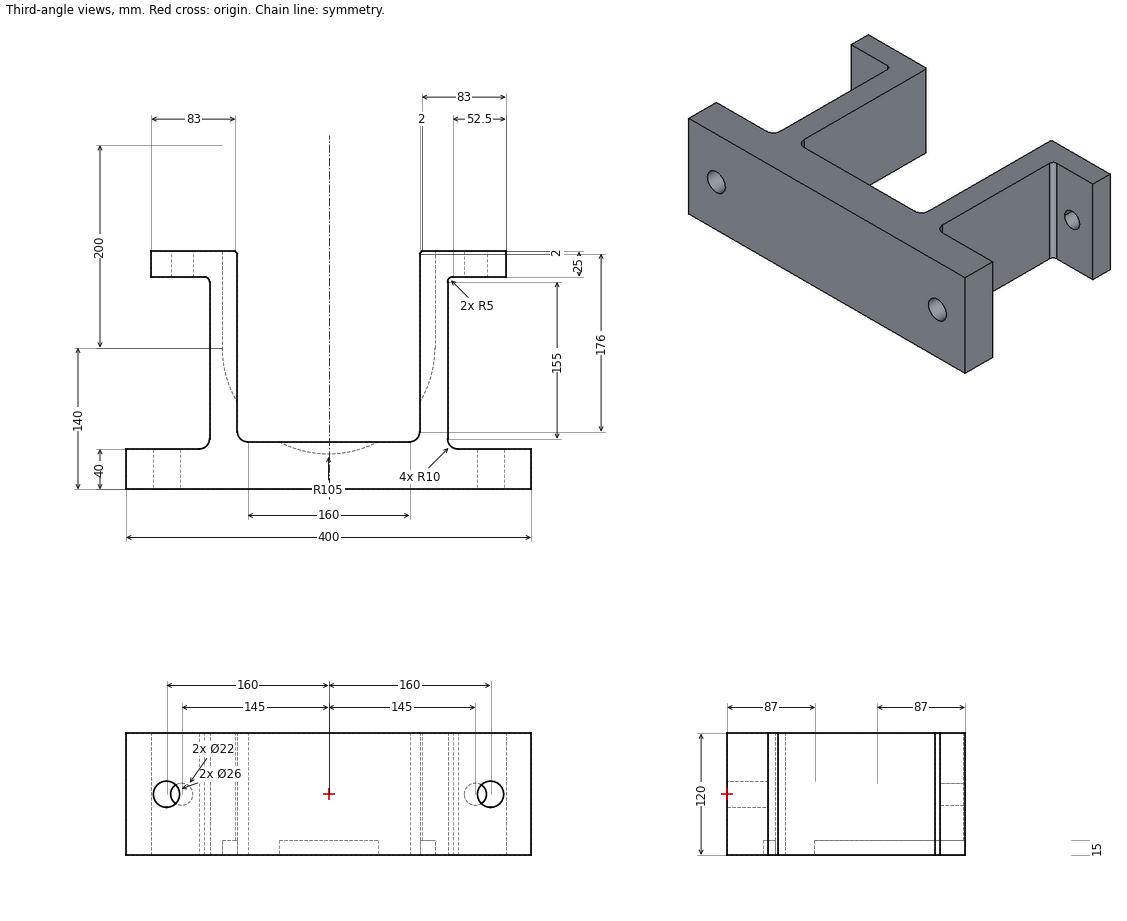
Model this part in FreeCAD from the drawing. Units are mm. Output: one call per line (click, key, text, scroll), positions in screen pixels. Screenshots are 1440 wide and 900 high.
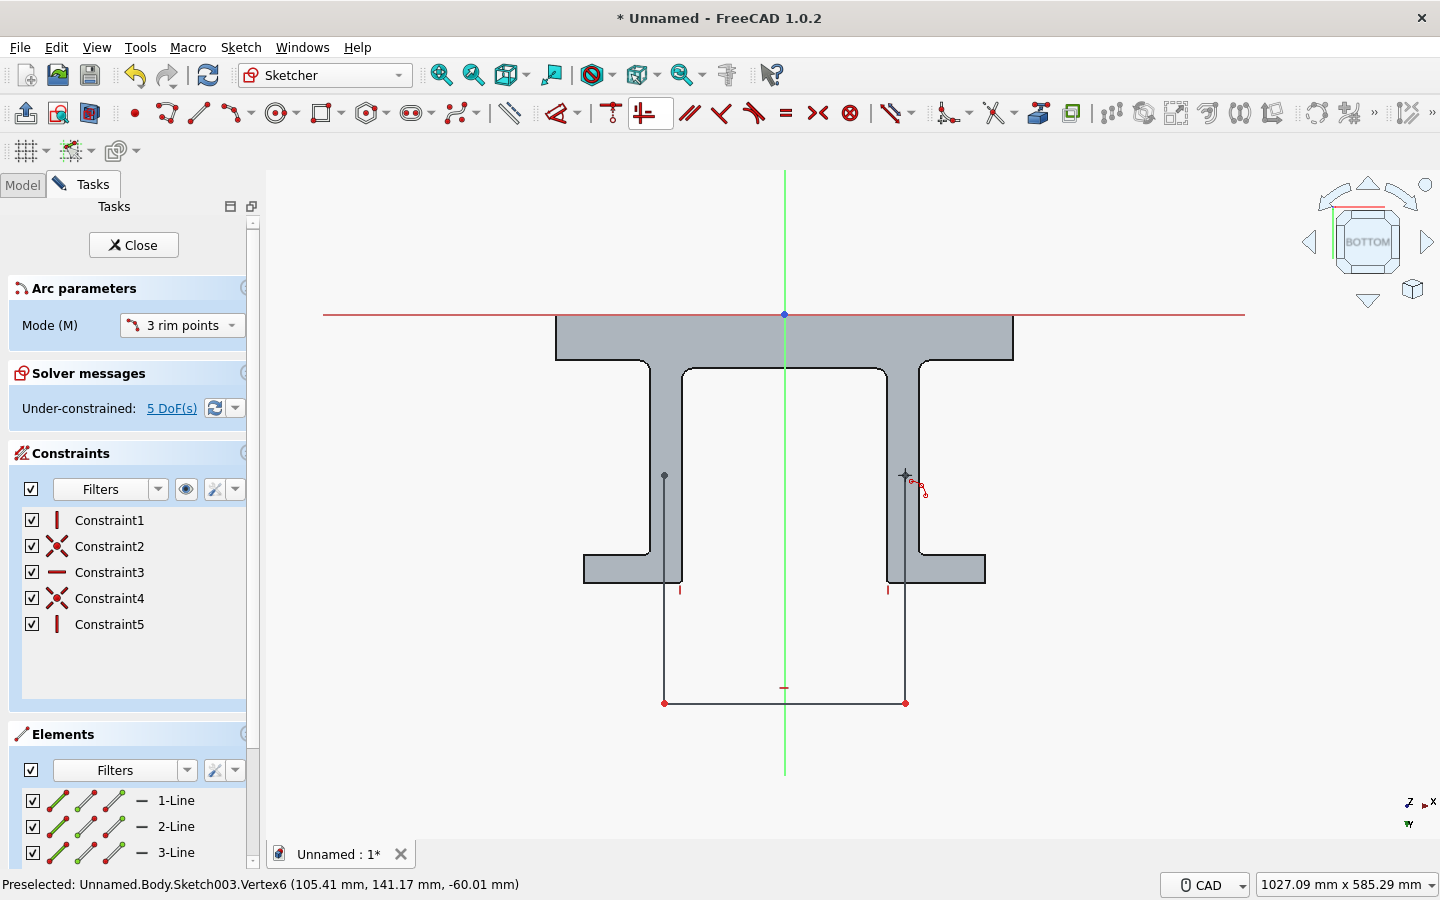
click(905, 476)
click(664, 476)
click(822, 361)
key(Escape)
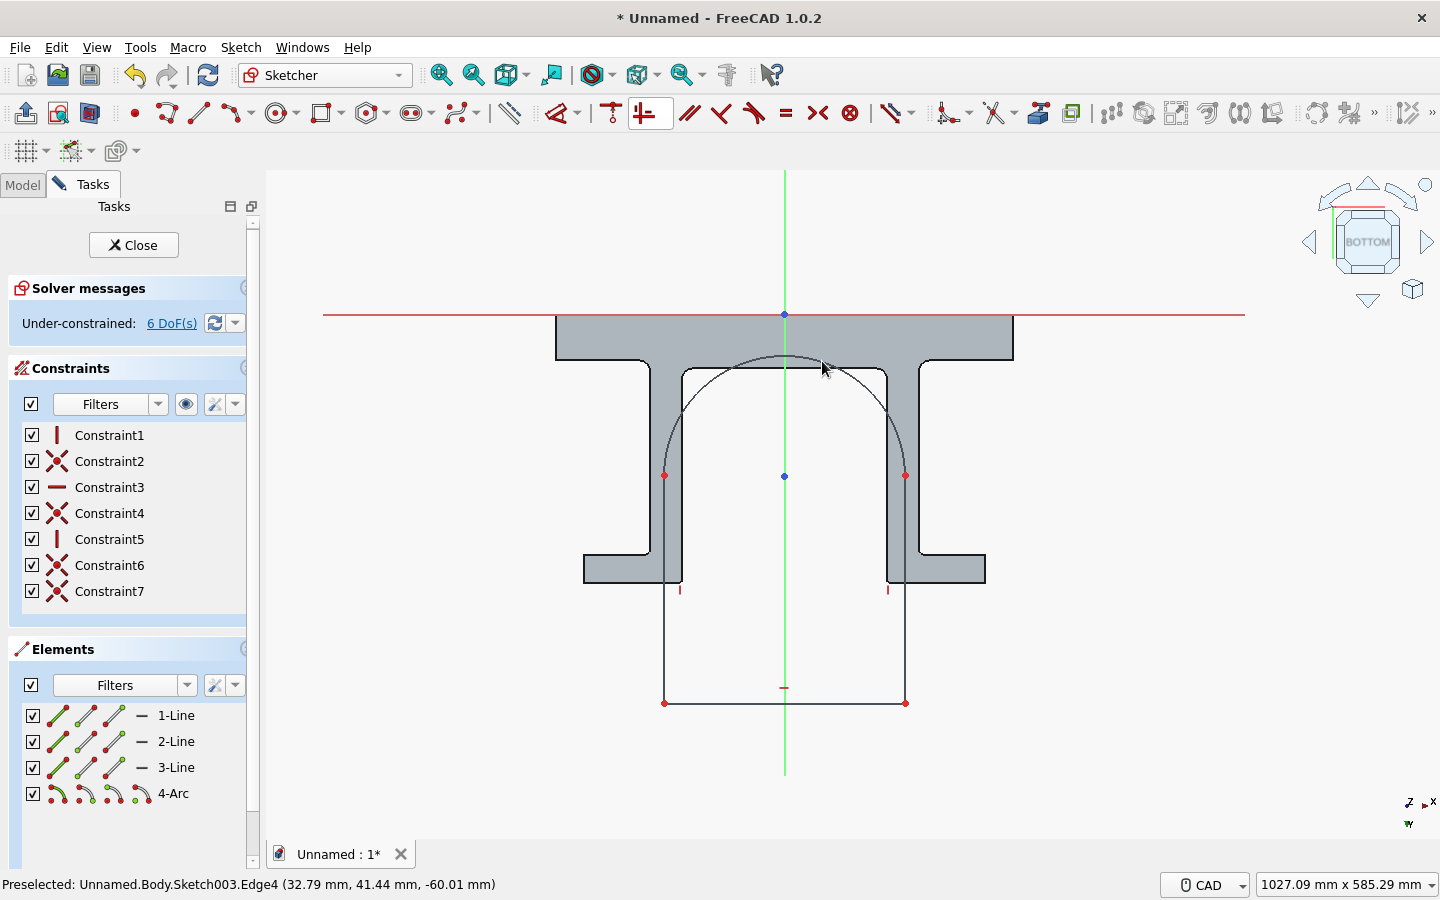
click(784, 477)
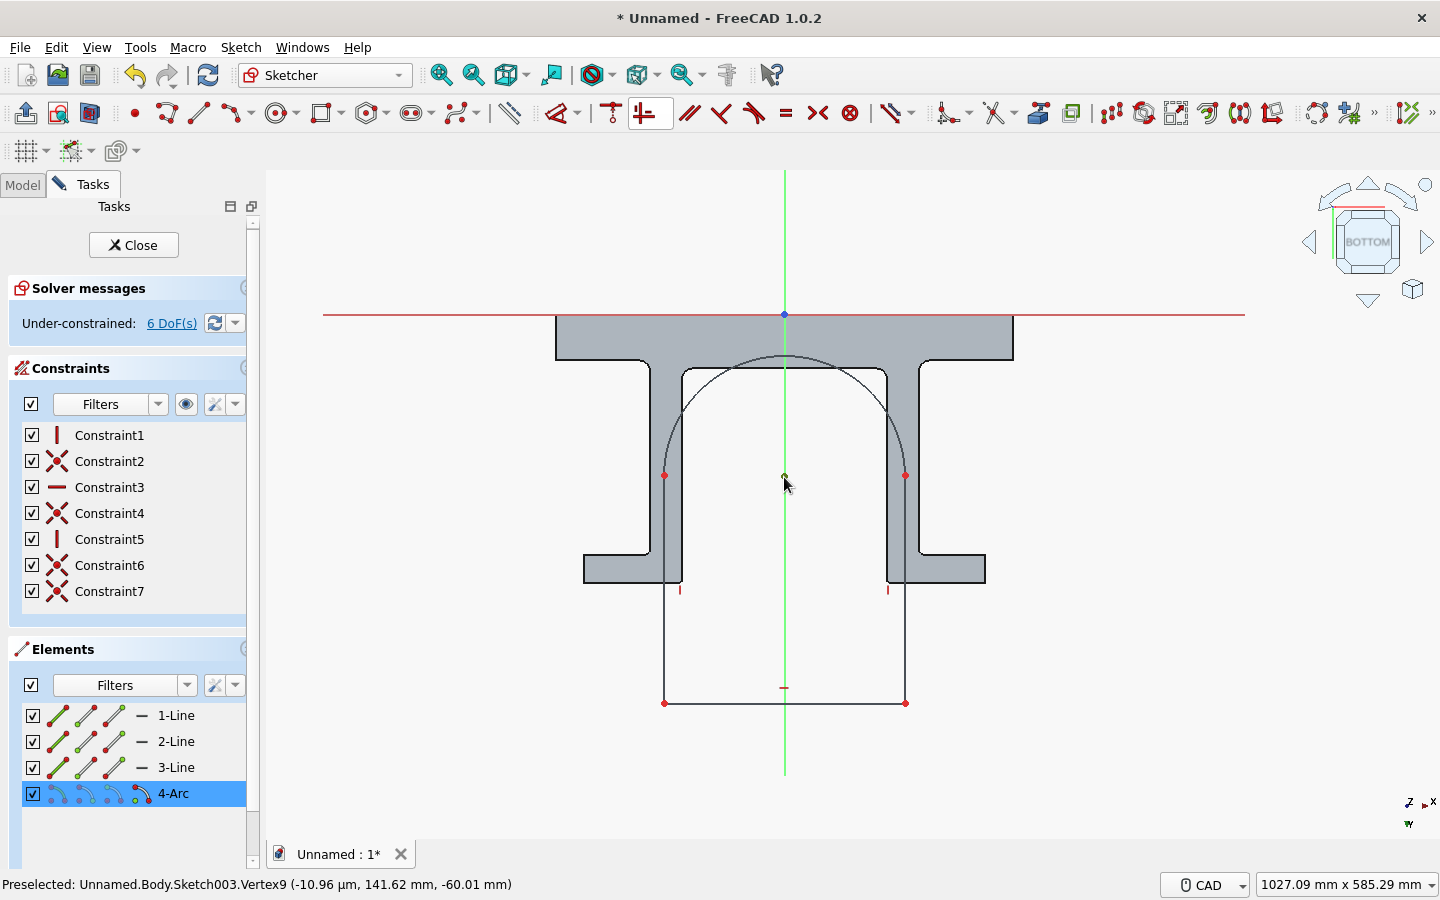
click(785, 767)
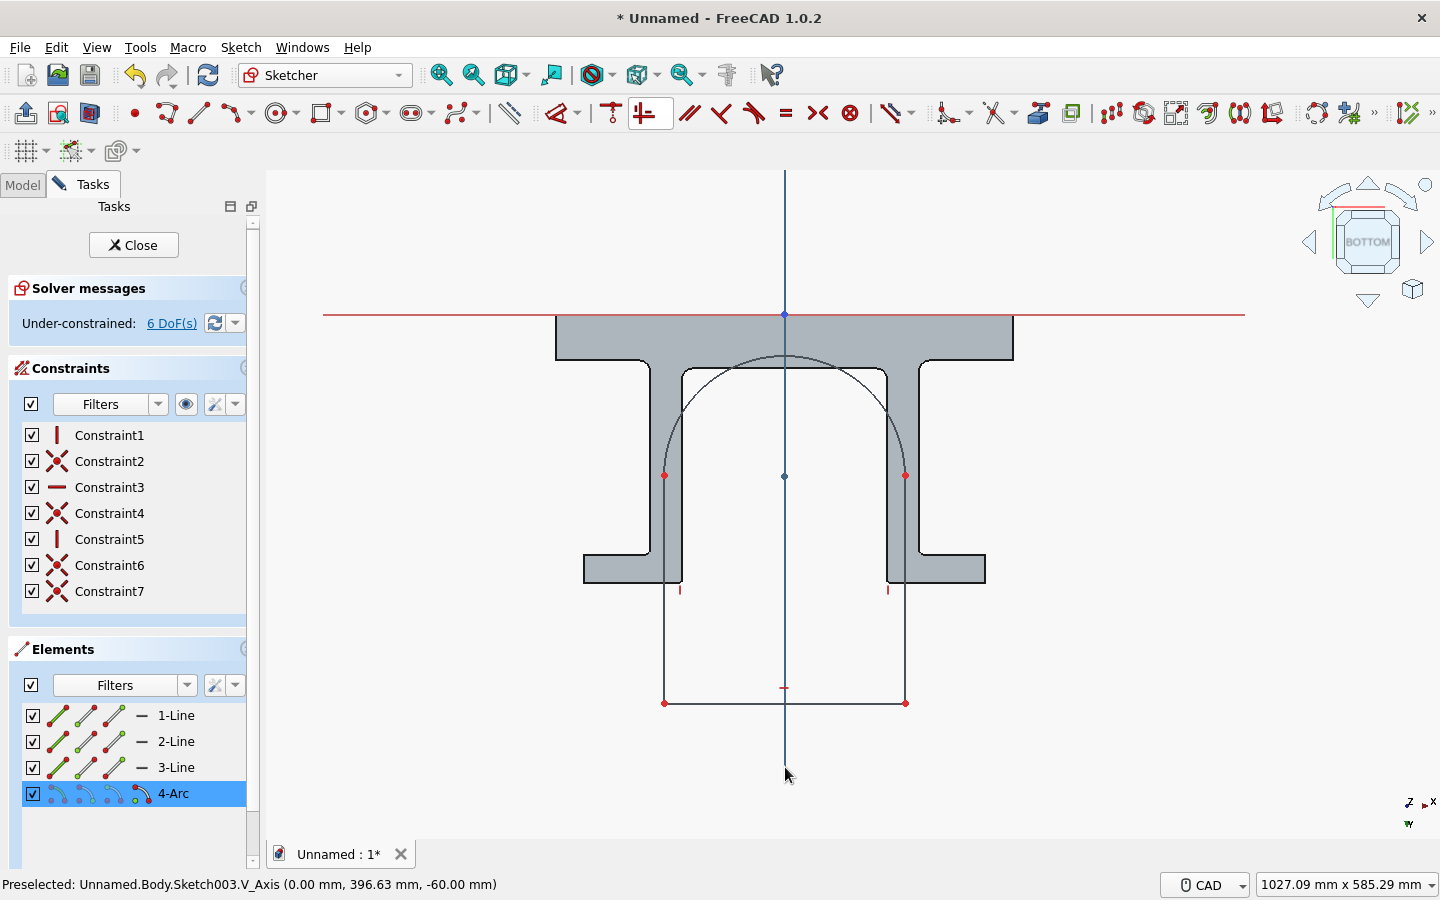
click(612, 114)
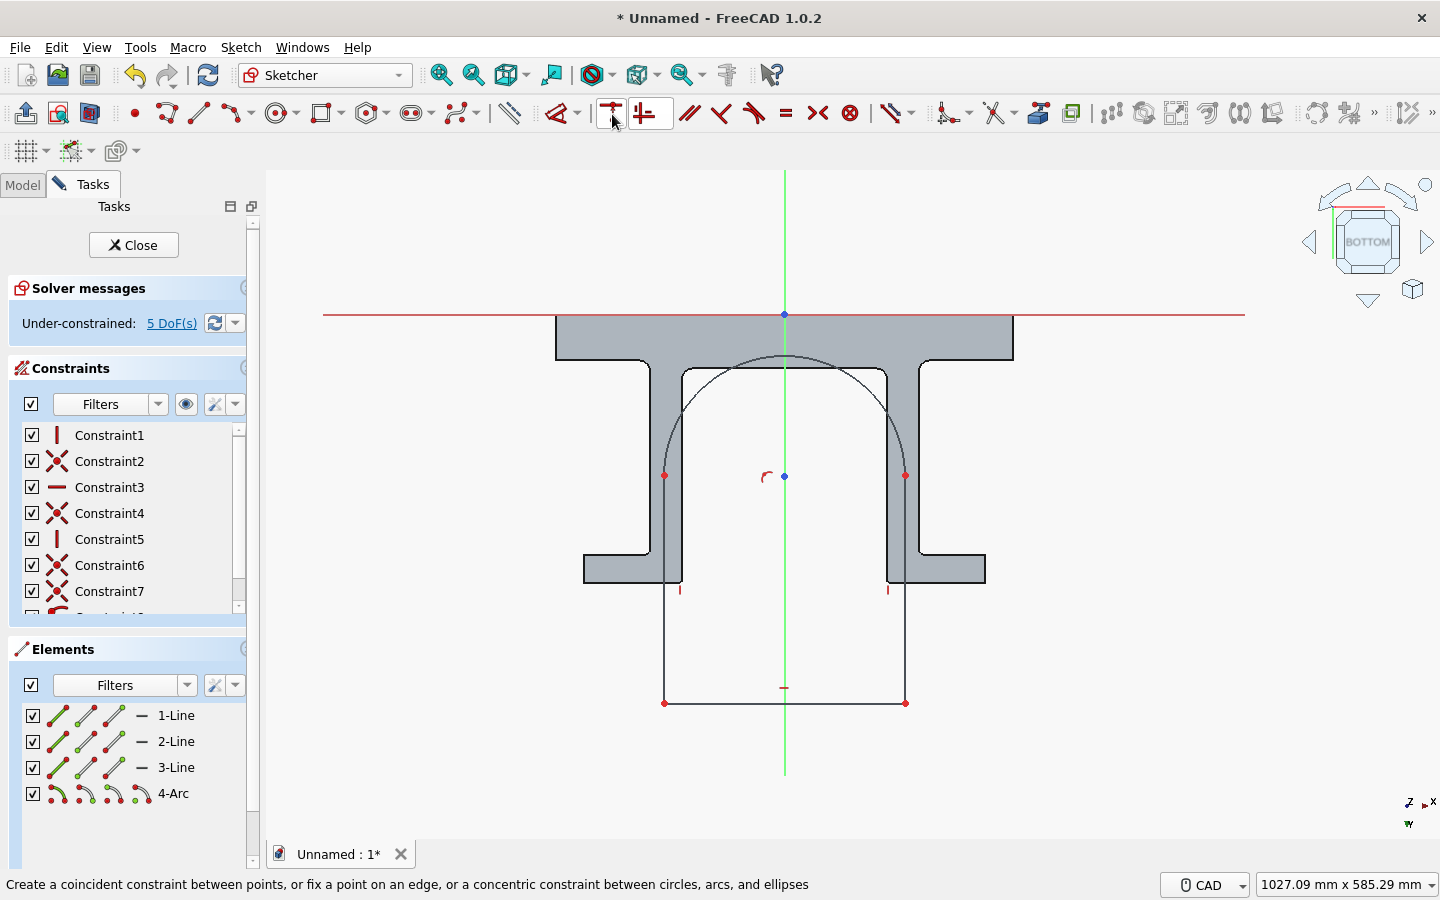
click(556, 114)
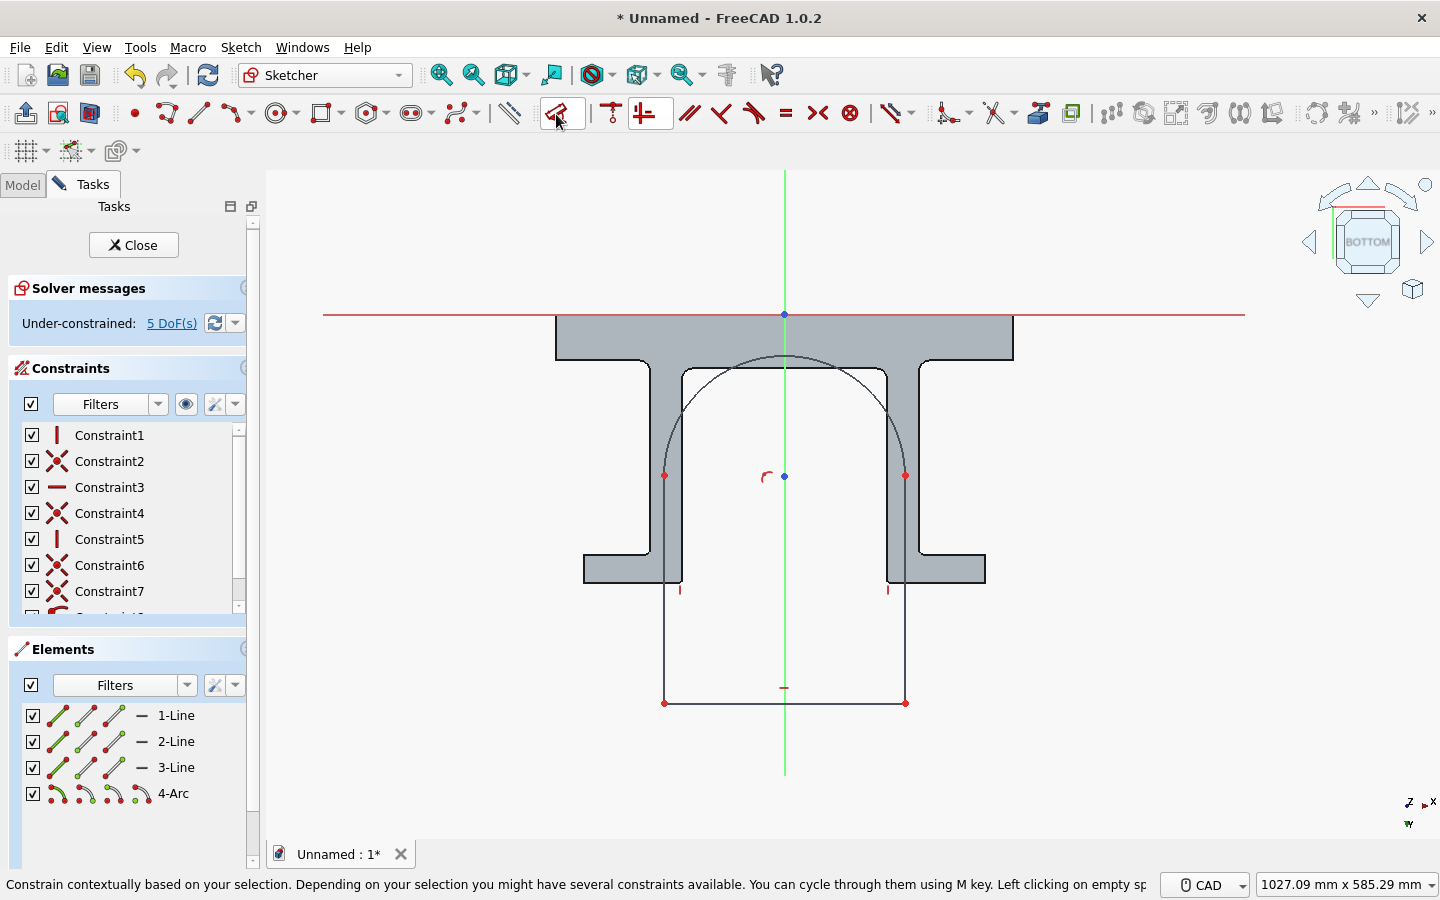
click(855, 379)
click(874, 353)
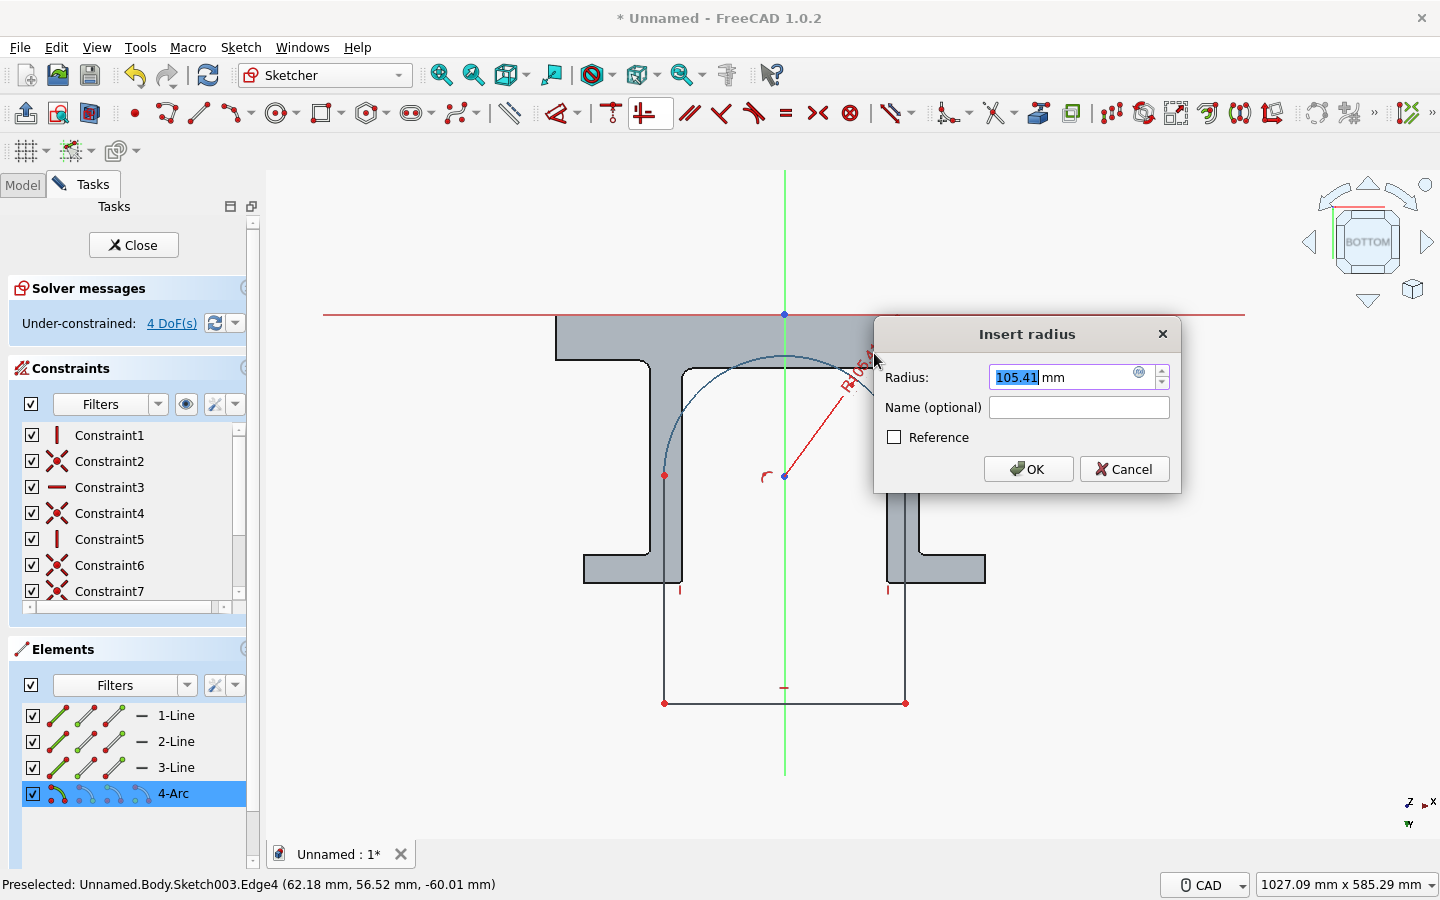
text(105)
key(Return)